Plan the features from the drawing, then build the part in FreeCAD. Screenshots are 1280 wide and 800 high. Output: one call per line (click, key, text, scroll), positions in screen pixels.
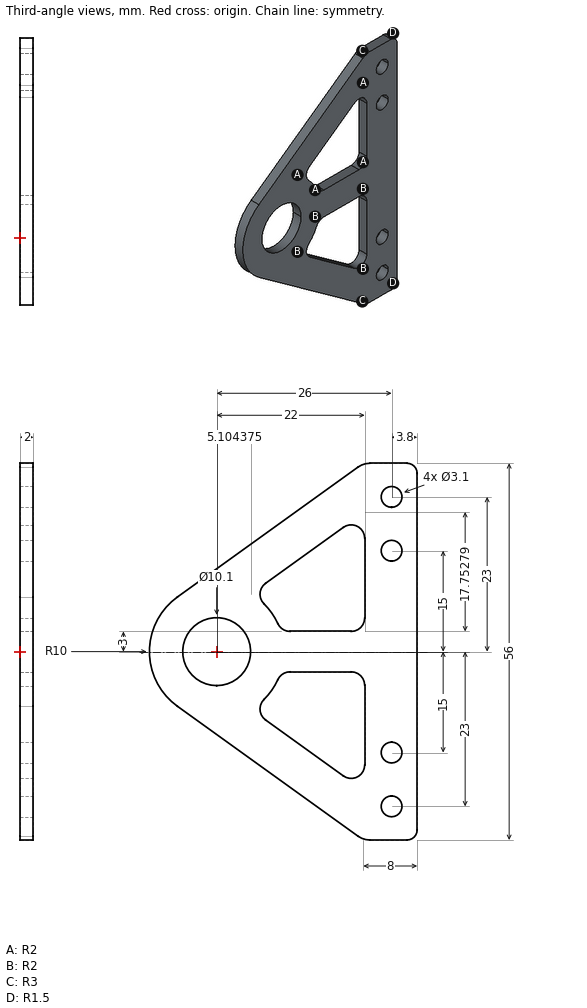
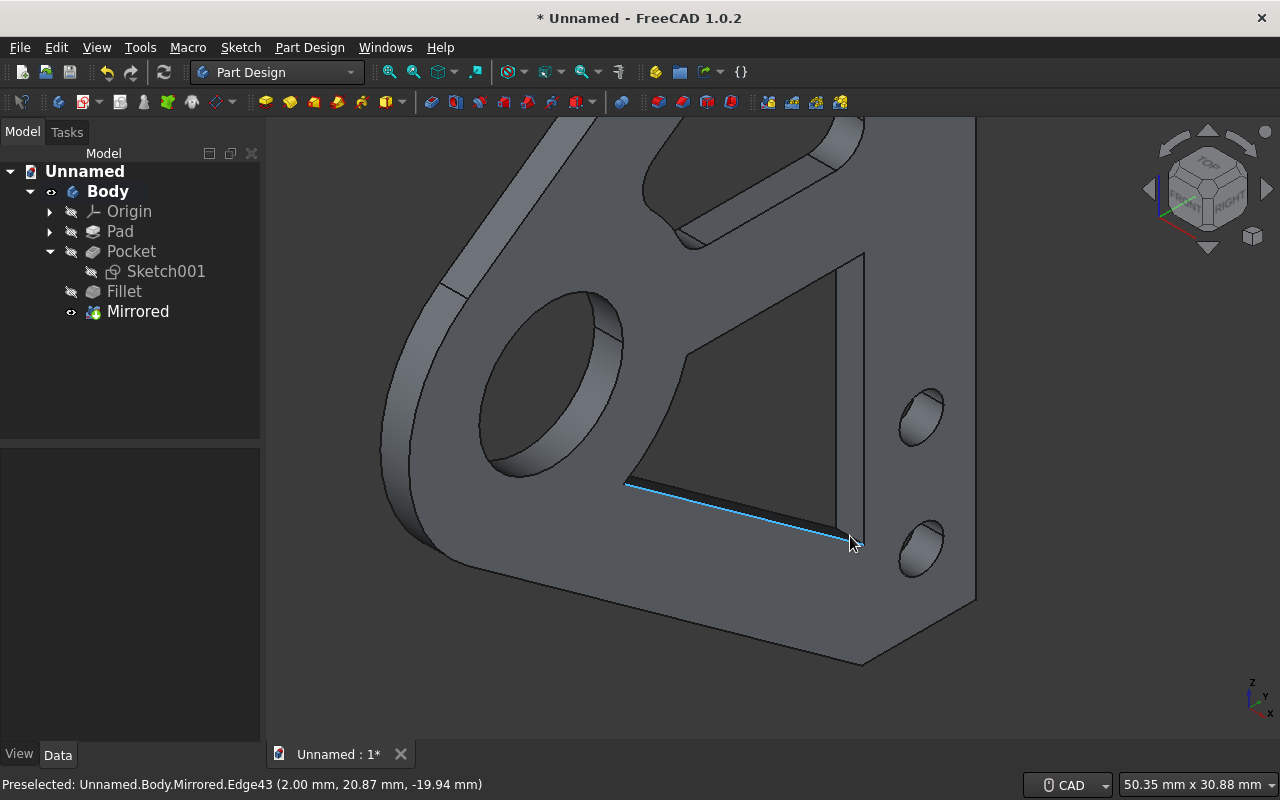
key(v)
key(f)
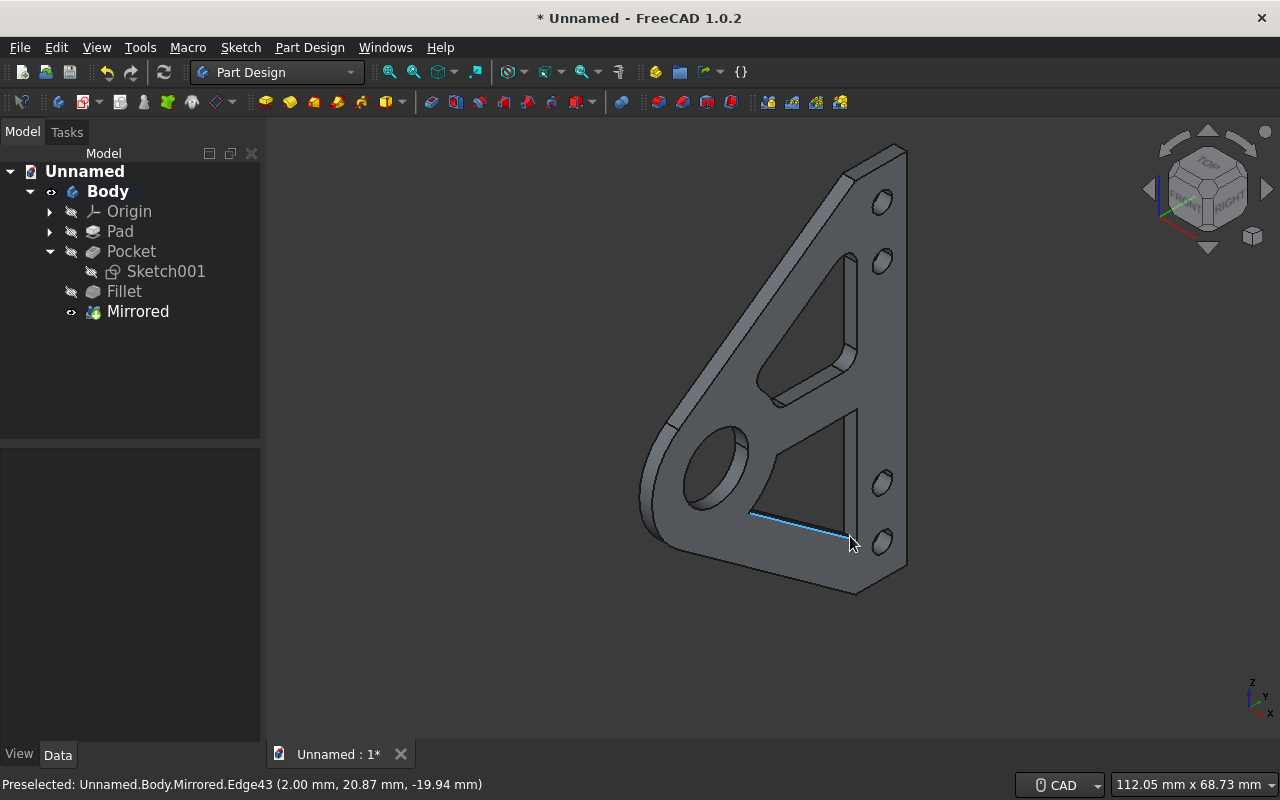
key(1)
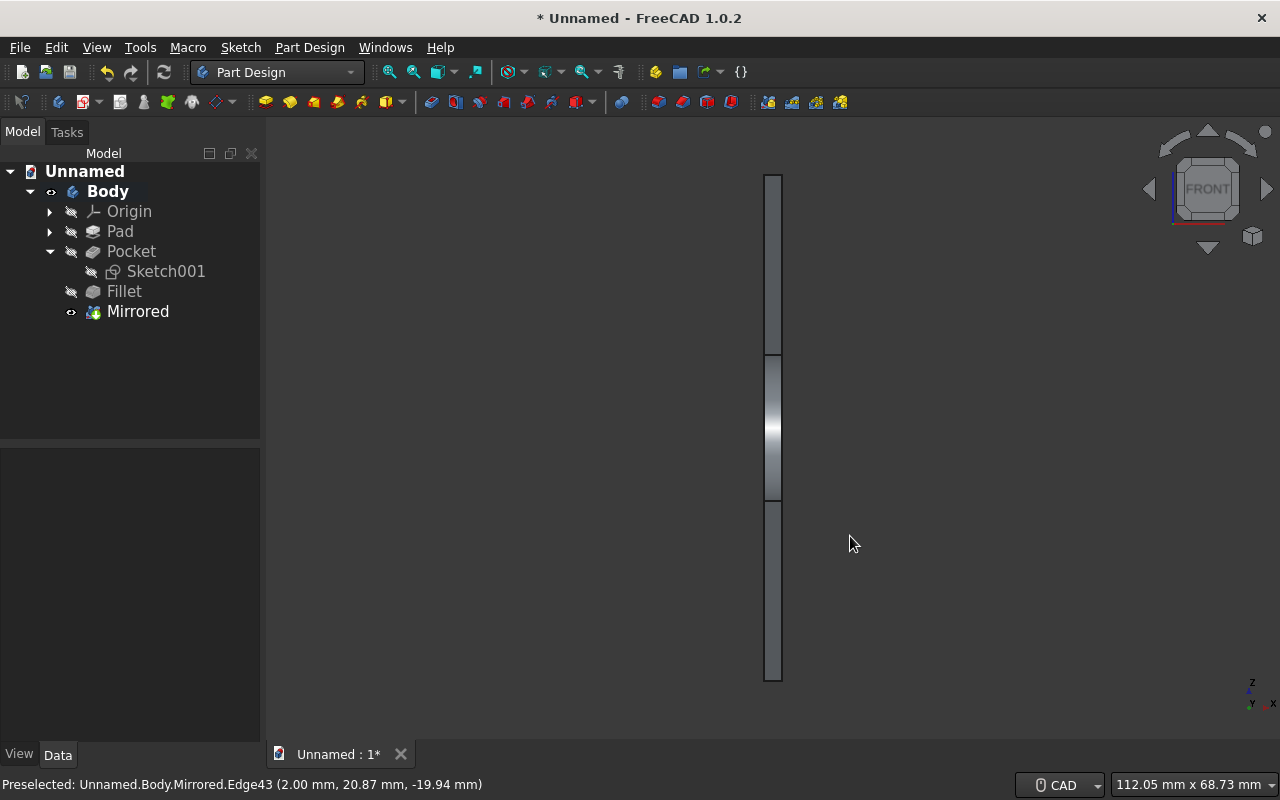
scroll(773, 615, up, 4)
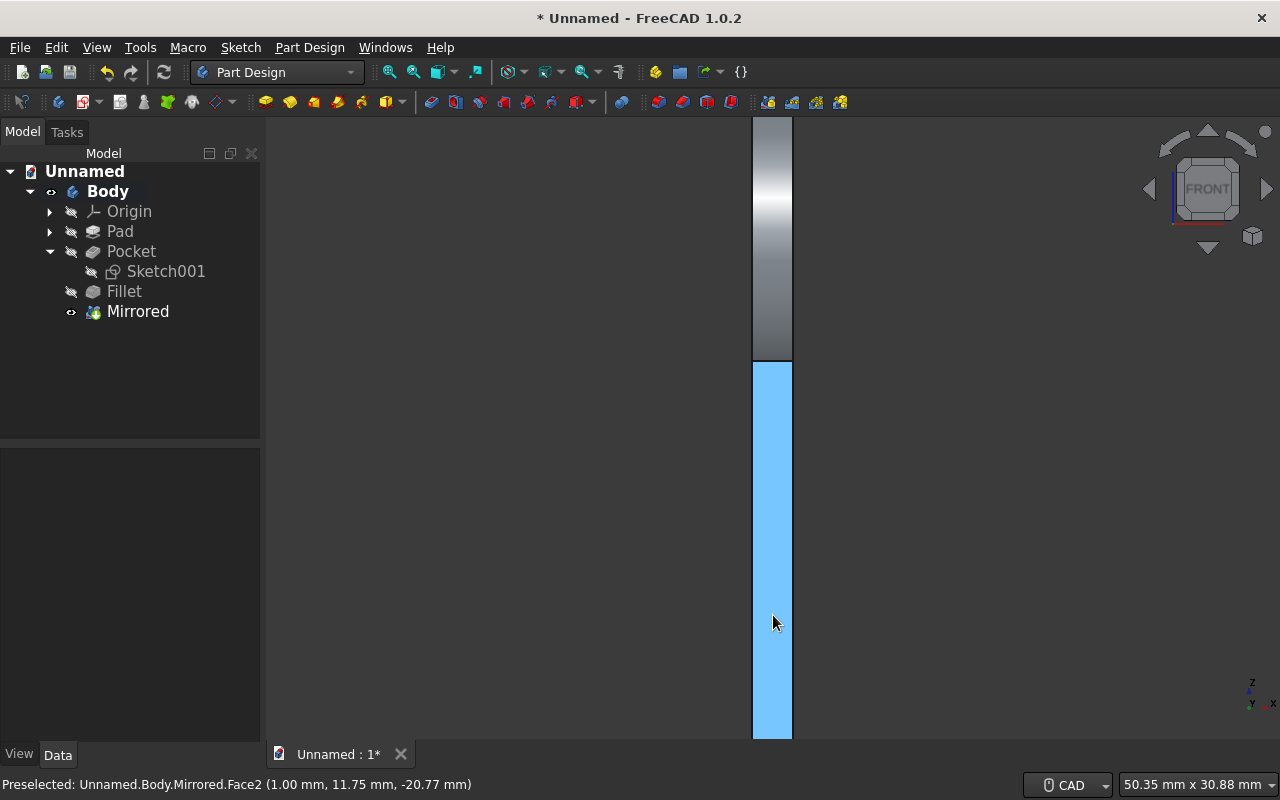
click(390, 72)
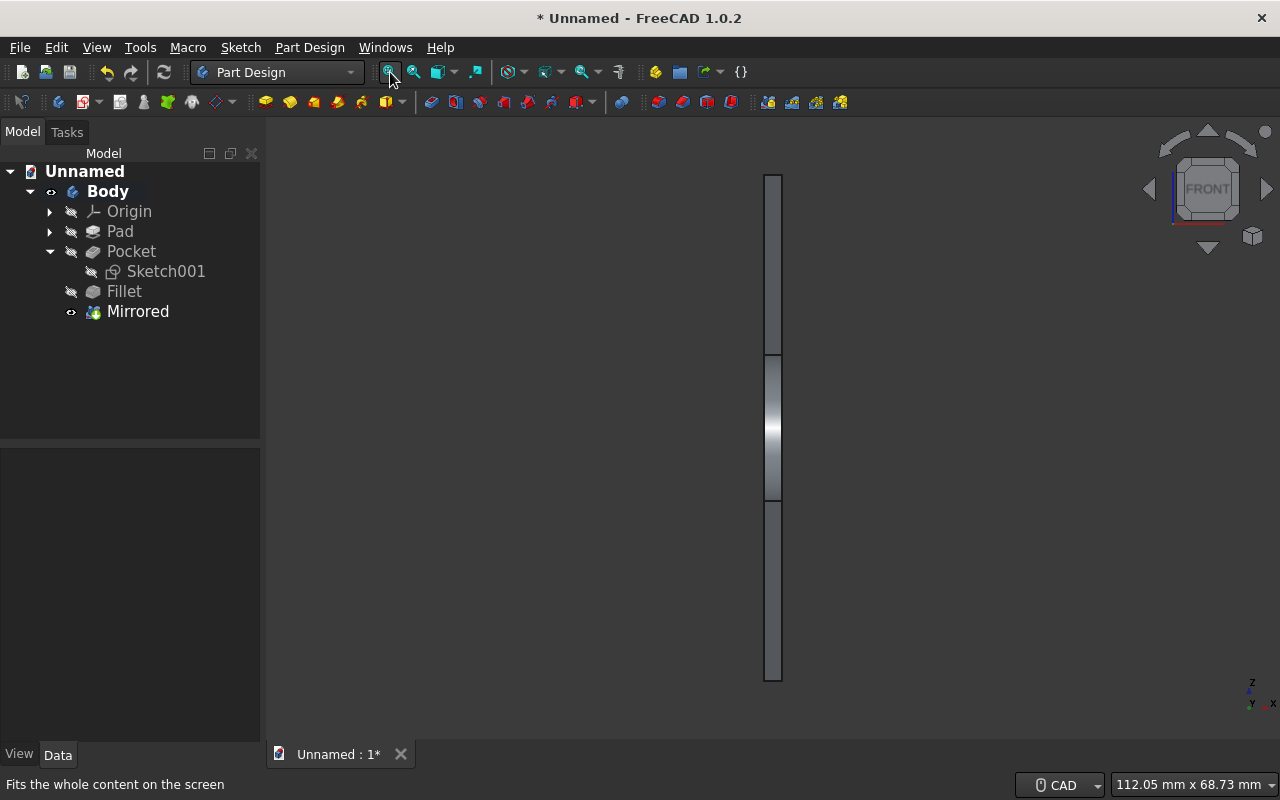
key(3)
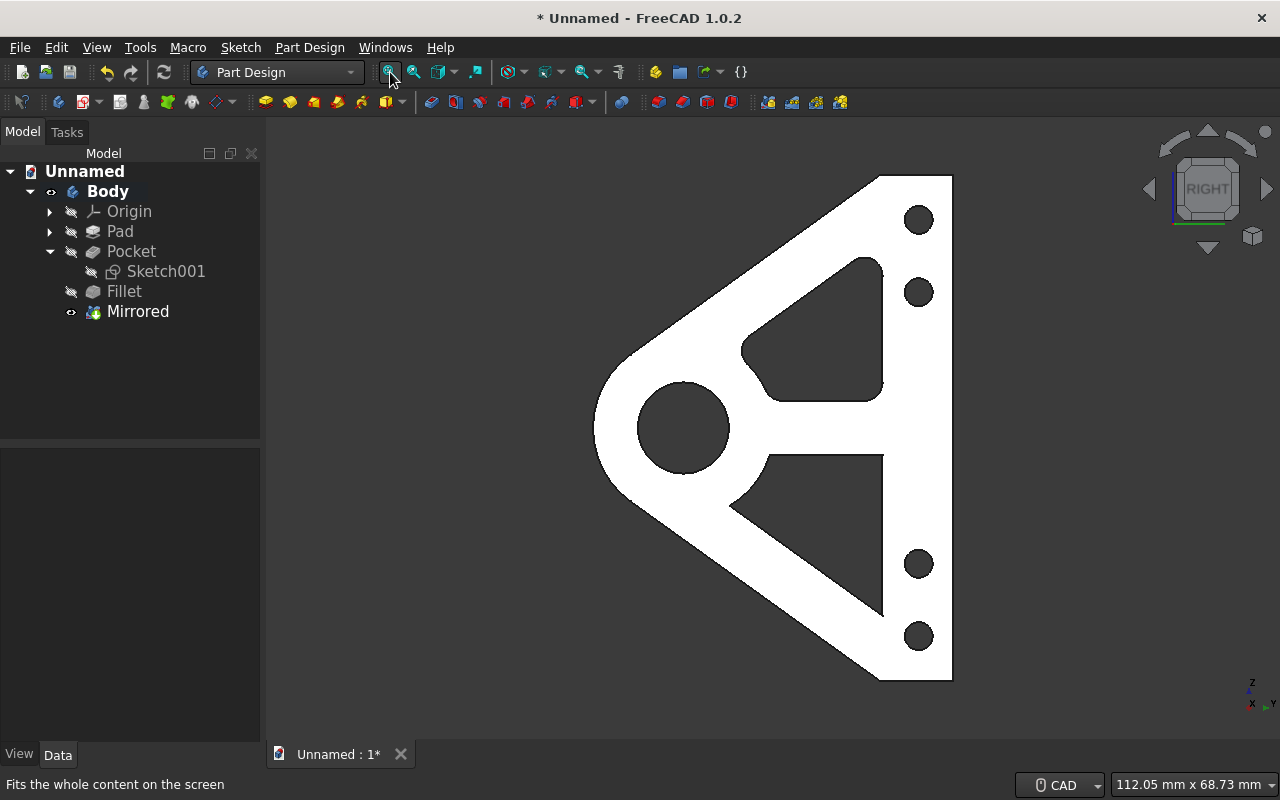
scroll(883, 615, up, 4)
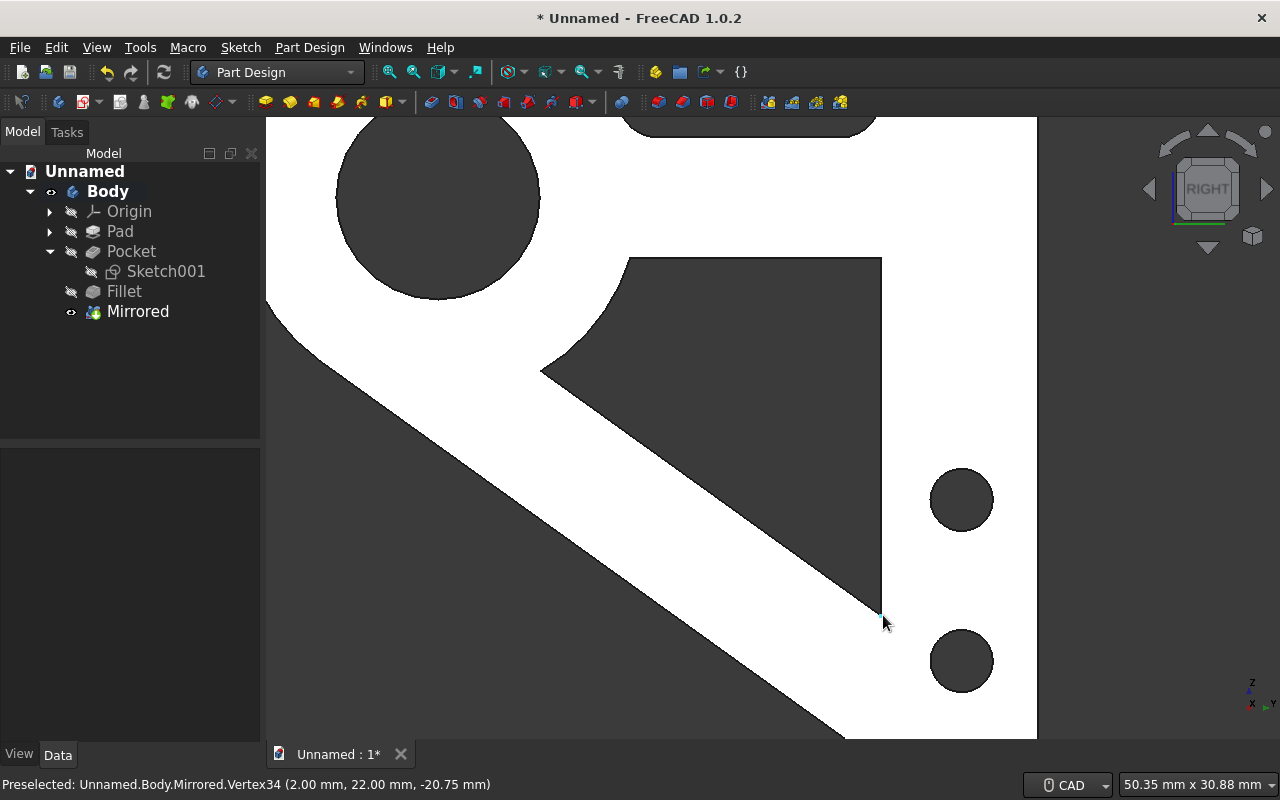
click(390, 72)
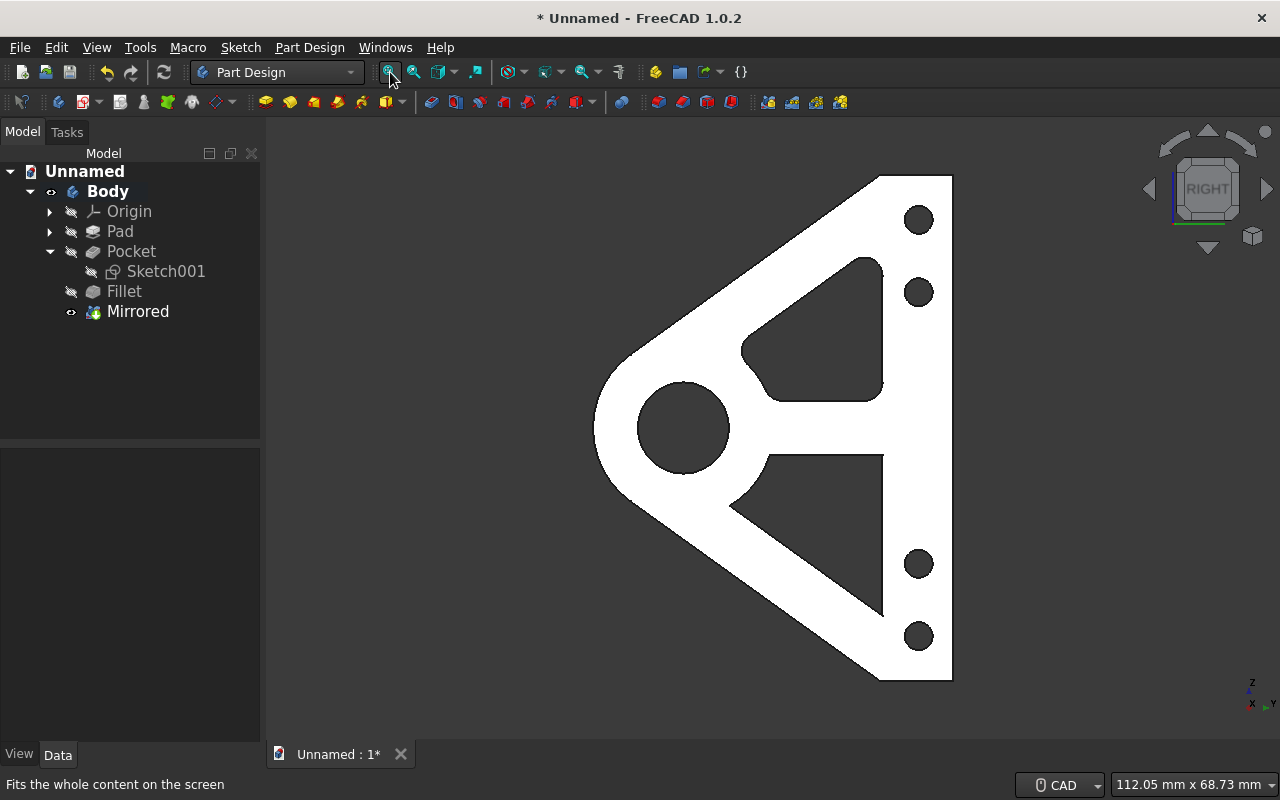
key(5)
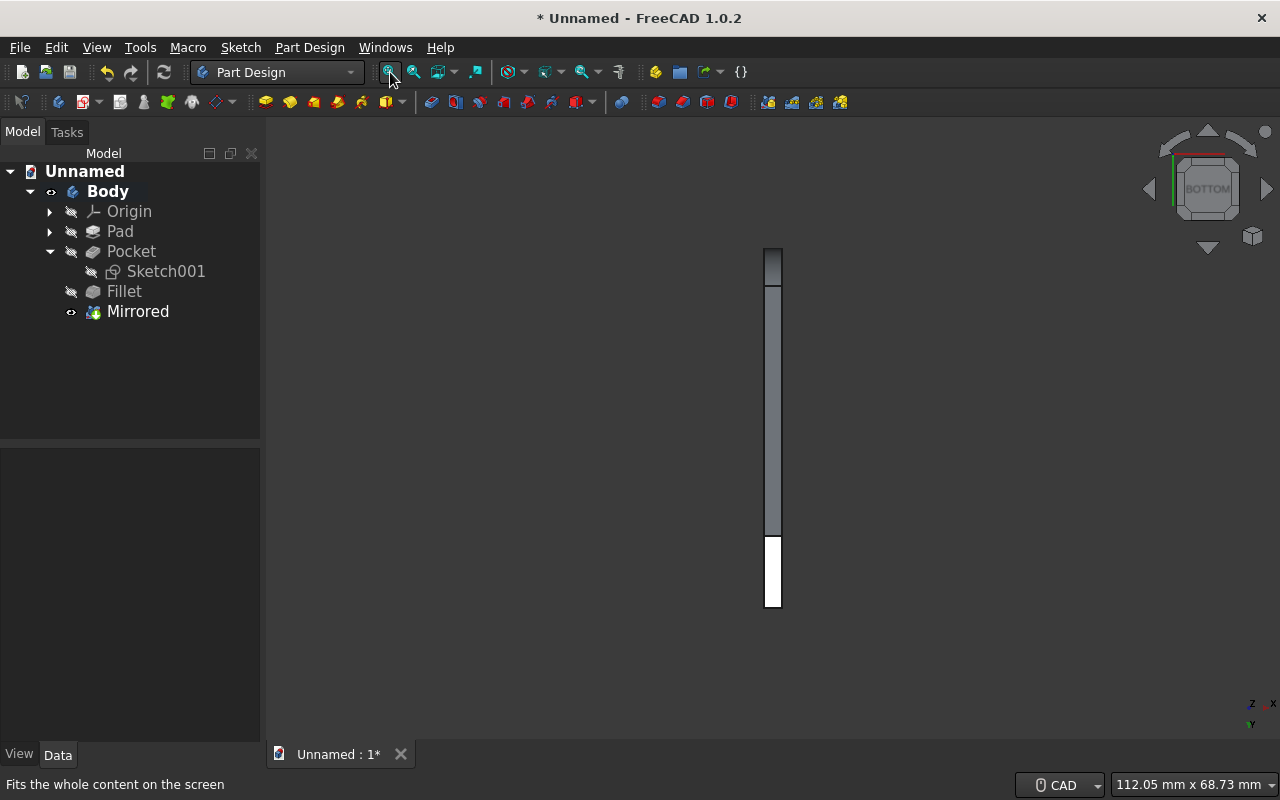
scroll(773, 537, up, 4)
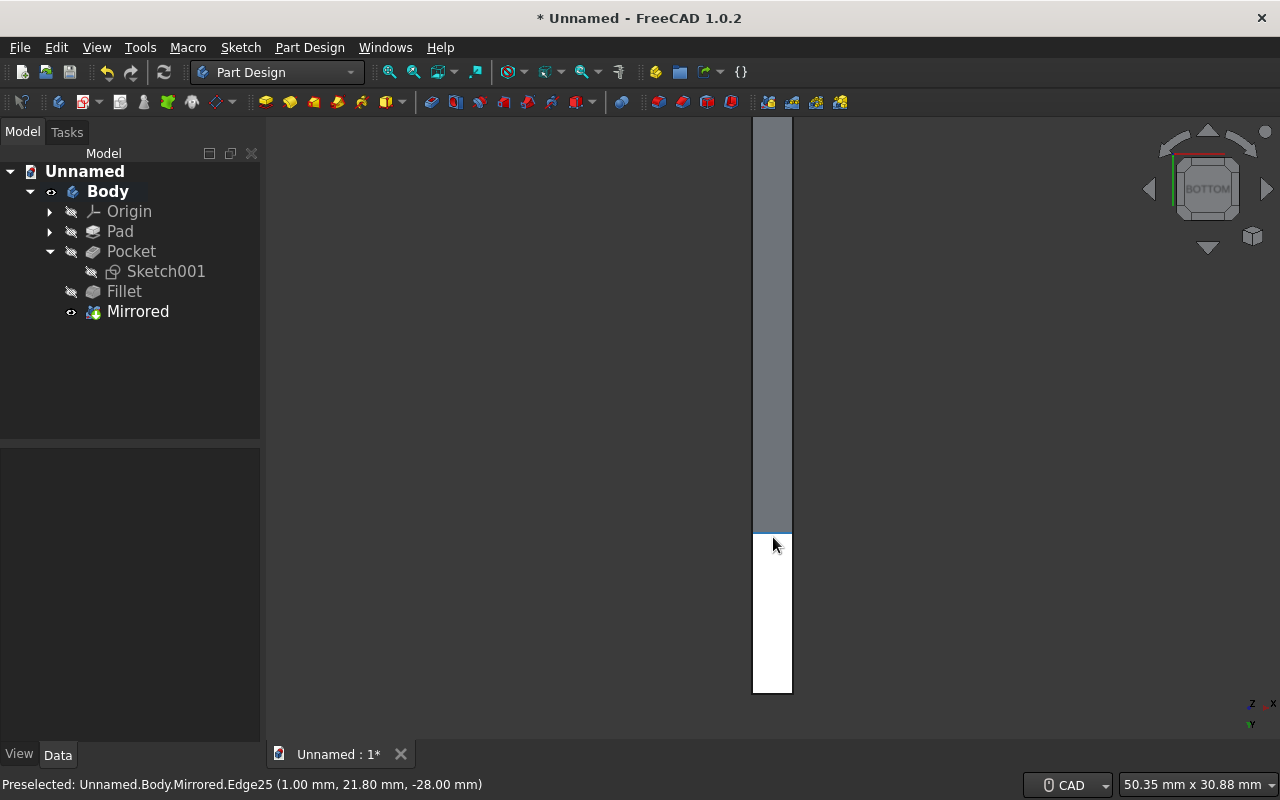
click(390, 72)